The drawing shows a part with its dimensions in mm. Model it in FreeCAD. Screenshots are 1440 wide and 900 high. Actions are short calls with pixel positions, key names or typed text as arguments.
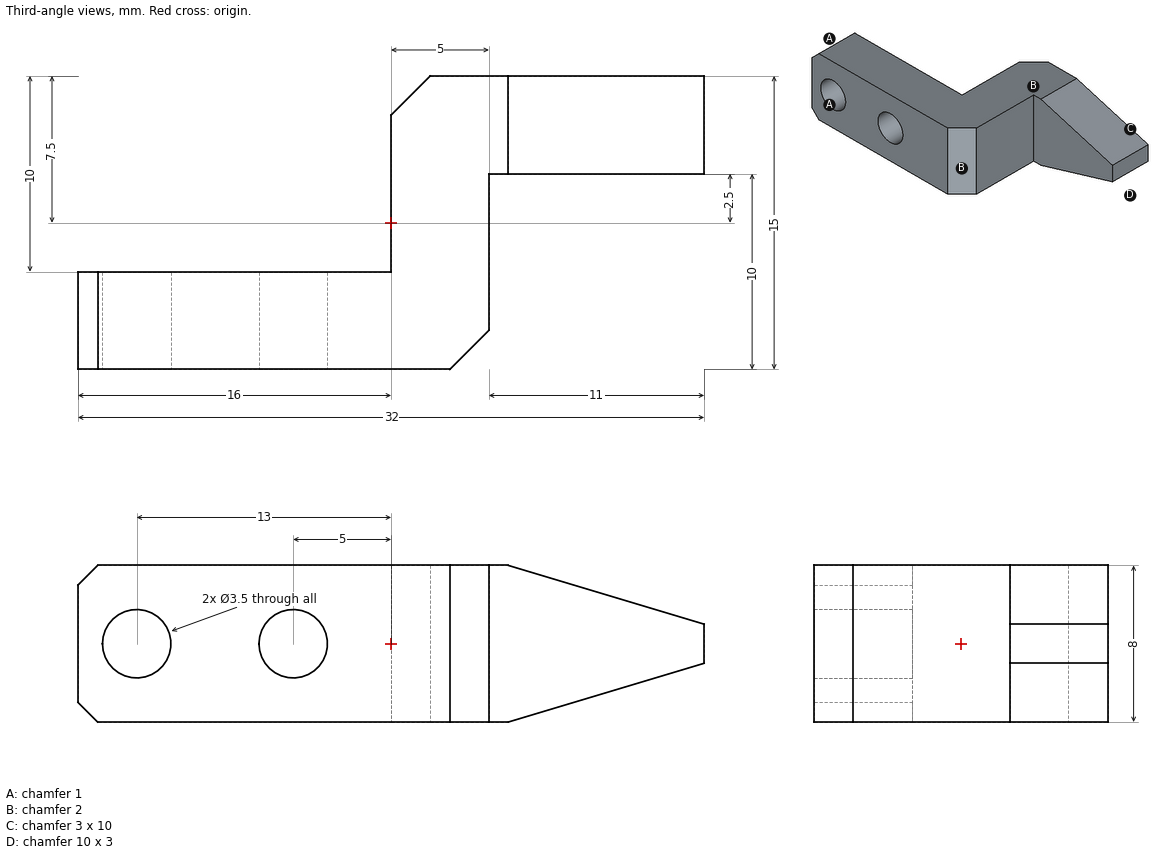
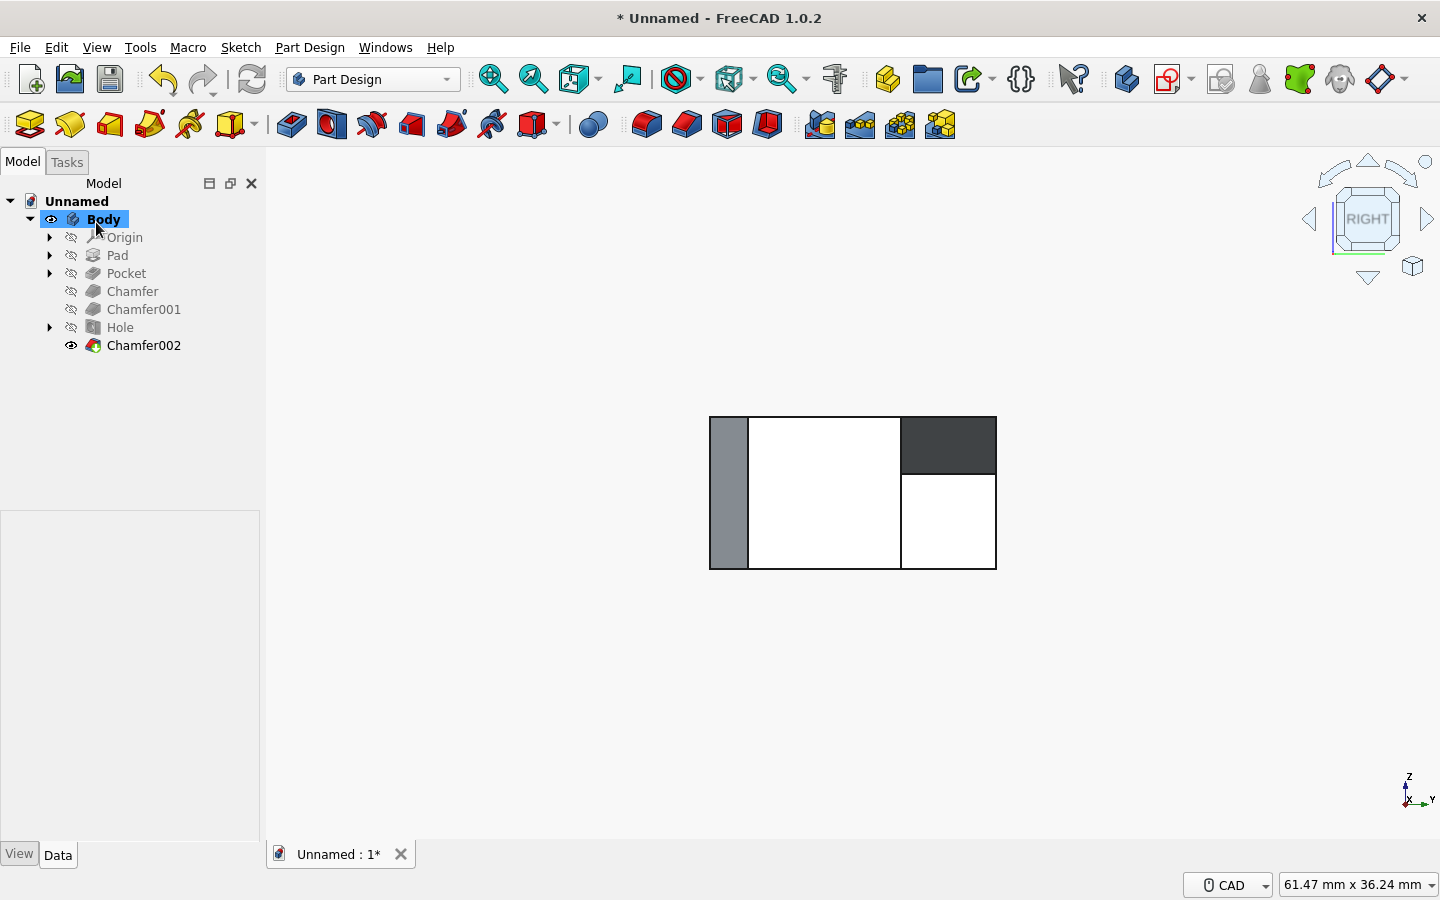
click(948, 568)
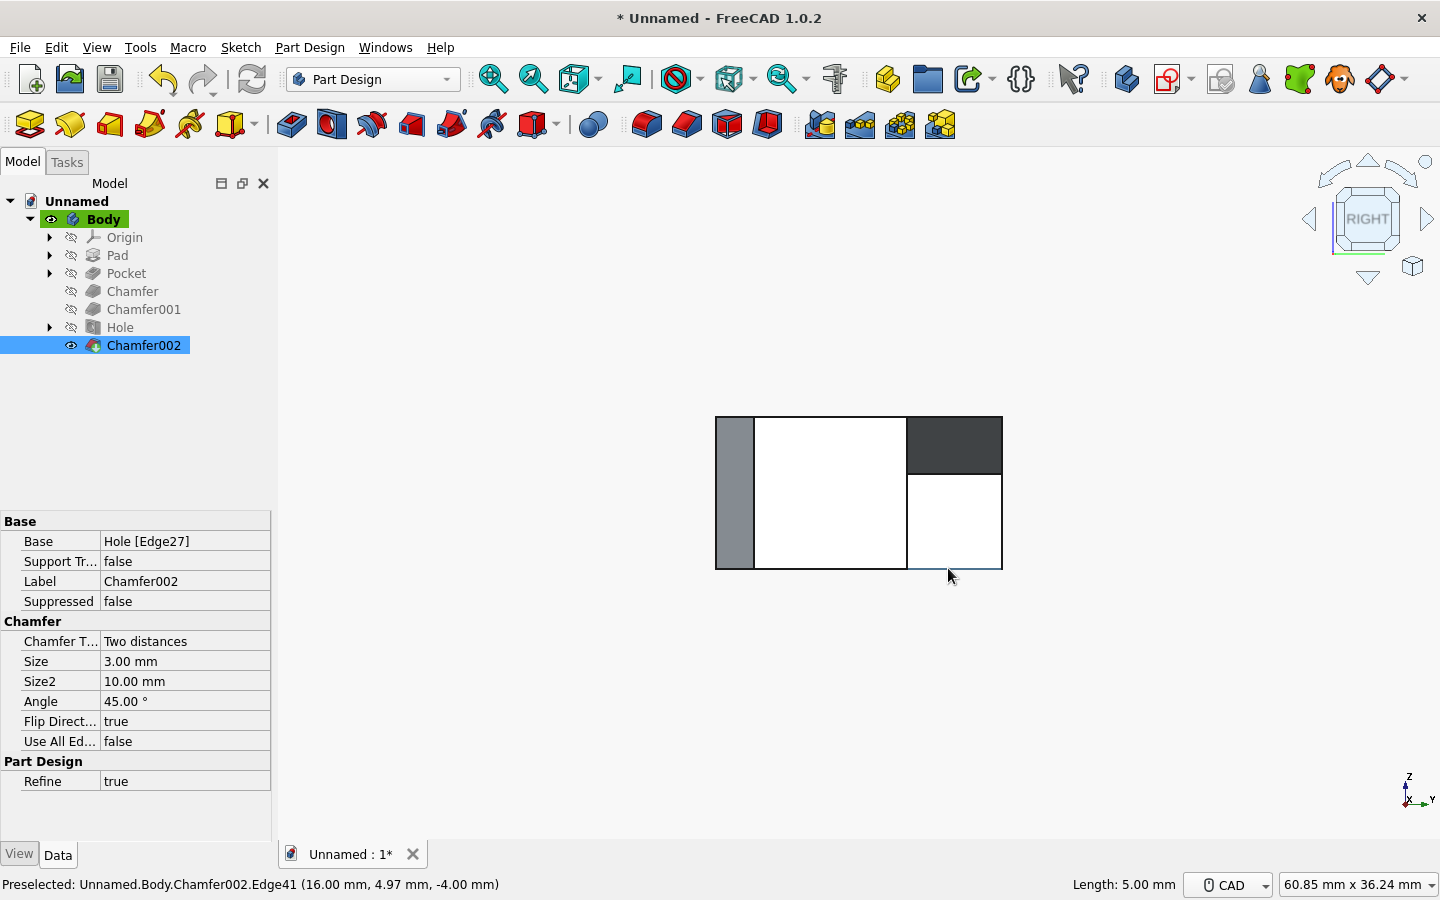
click(688, 124)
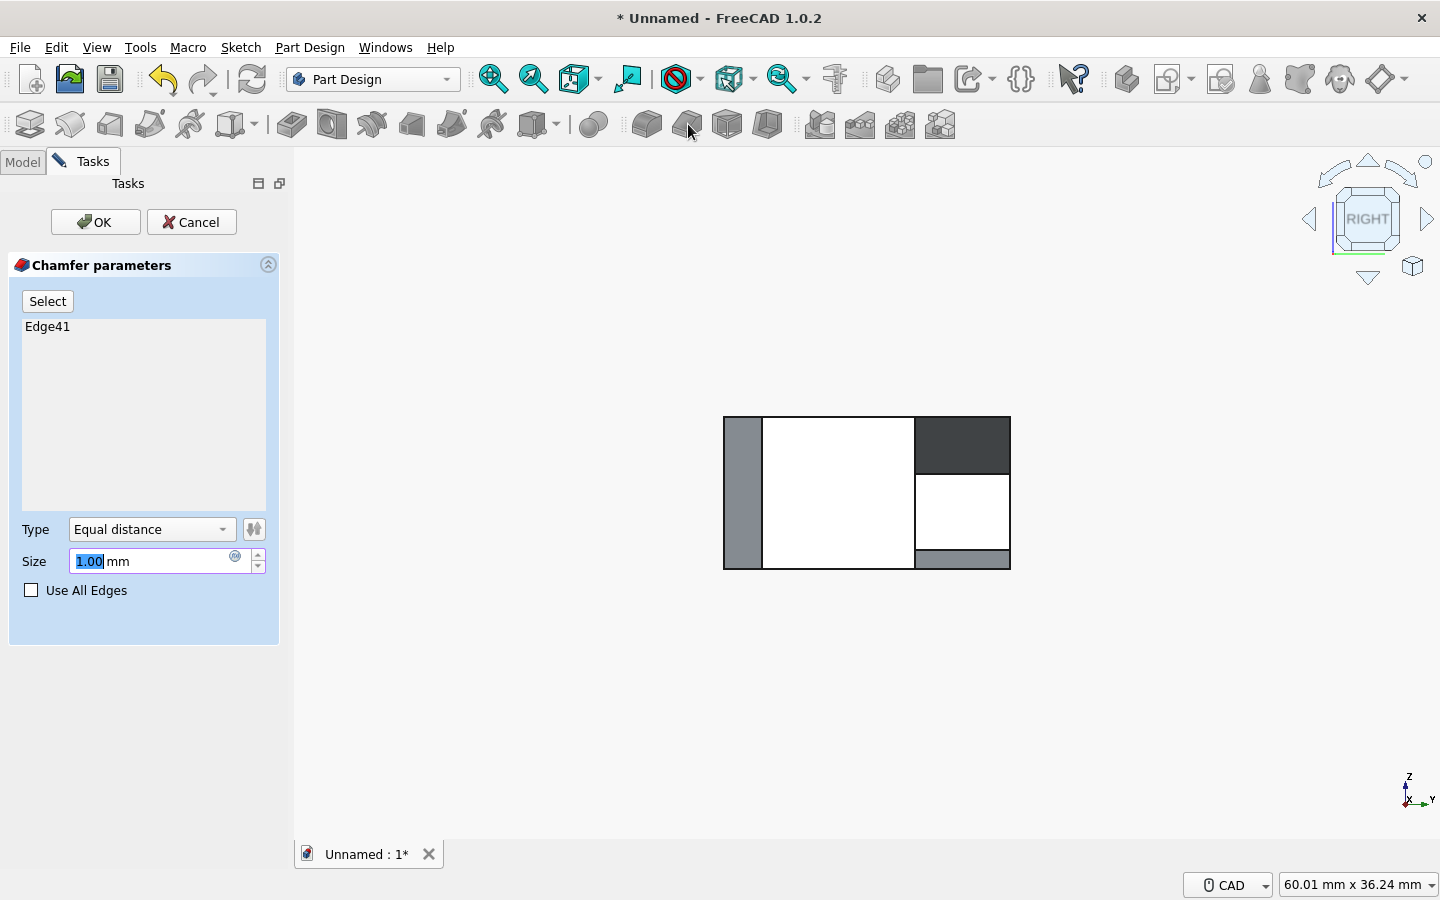
text(10)
key(Tab)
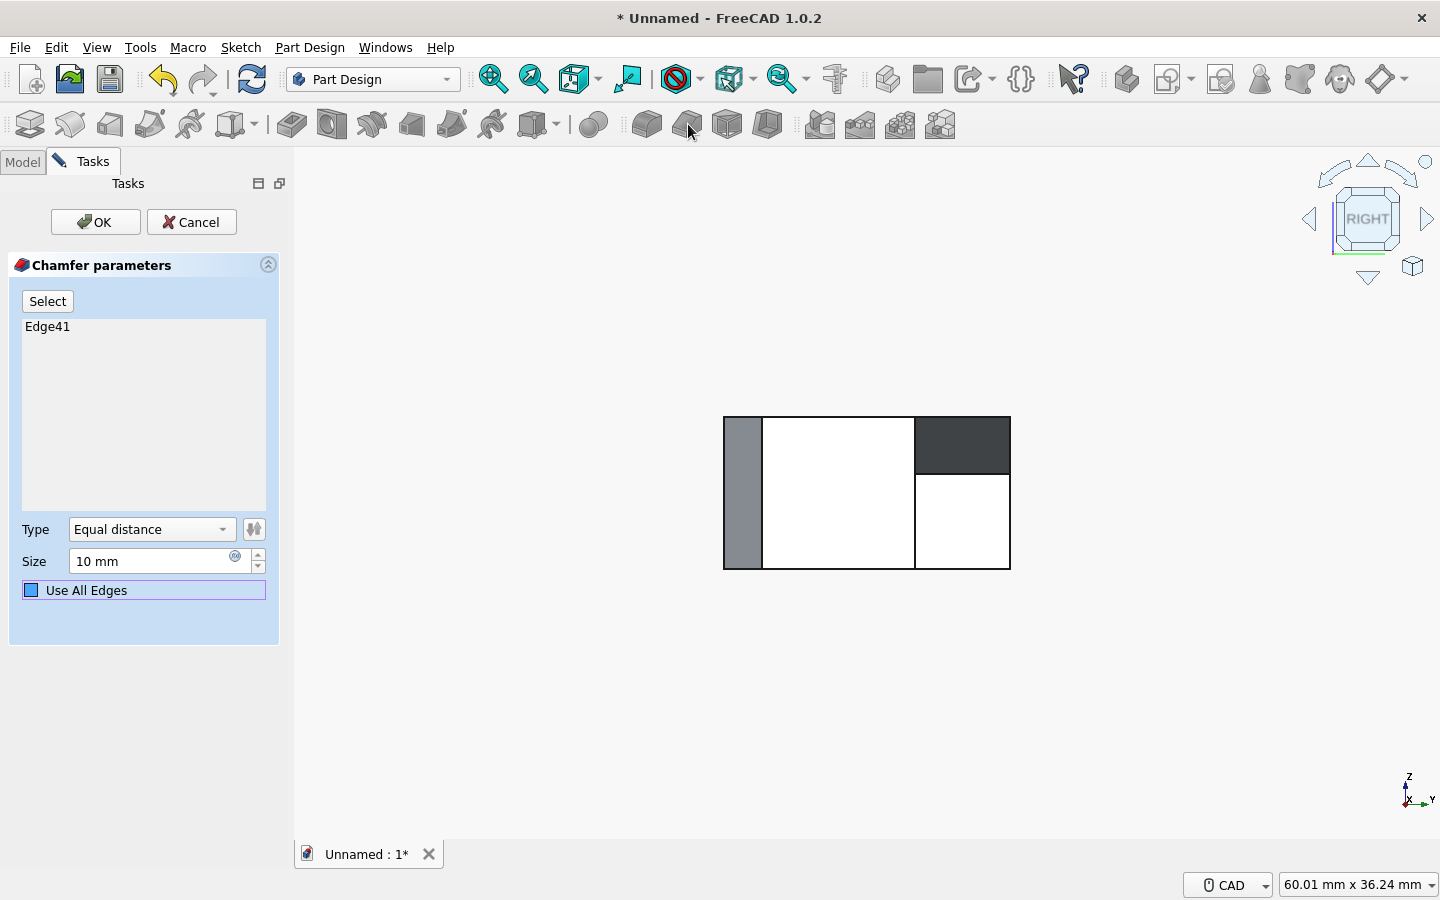
click(153, 530)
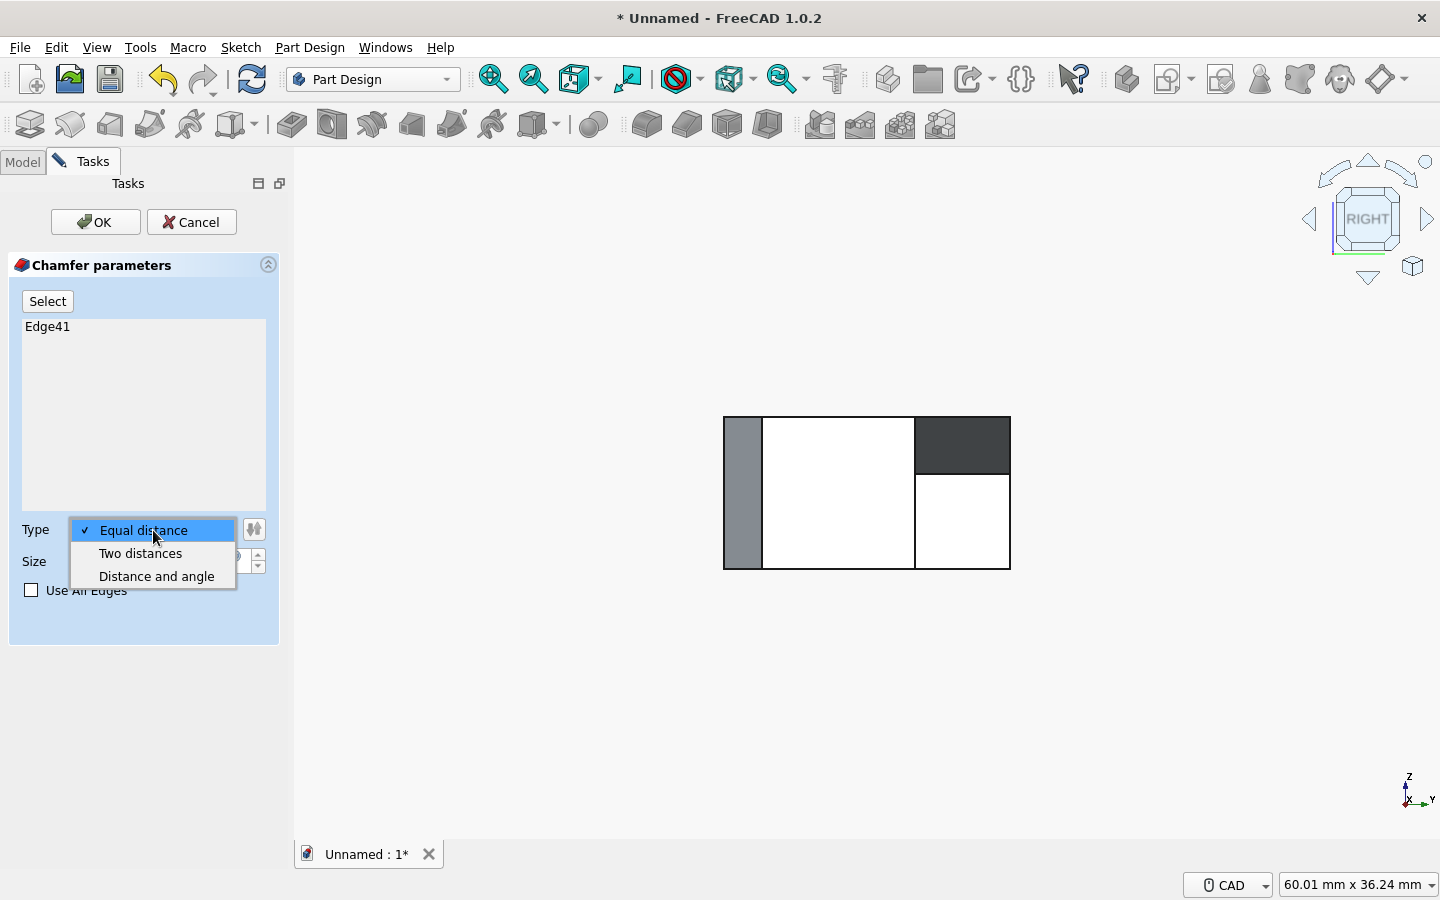
click(152, 554)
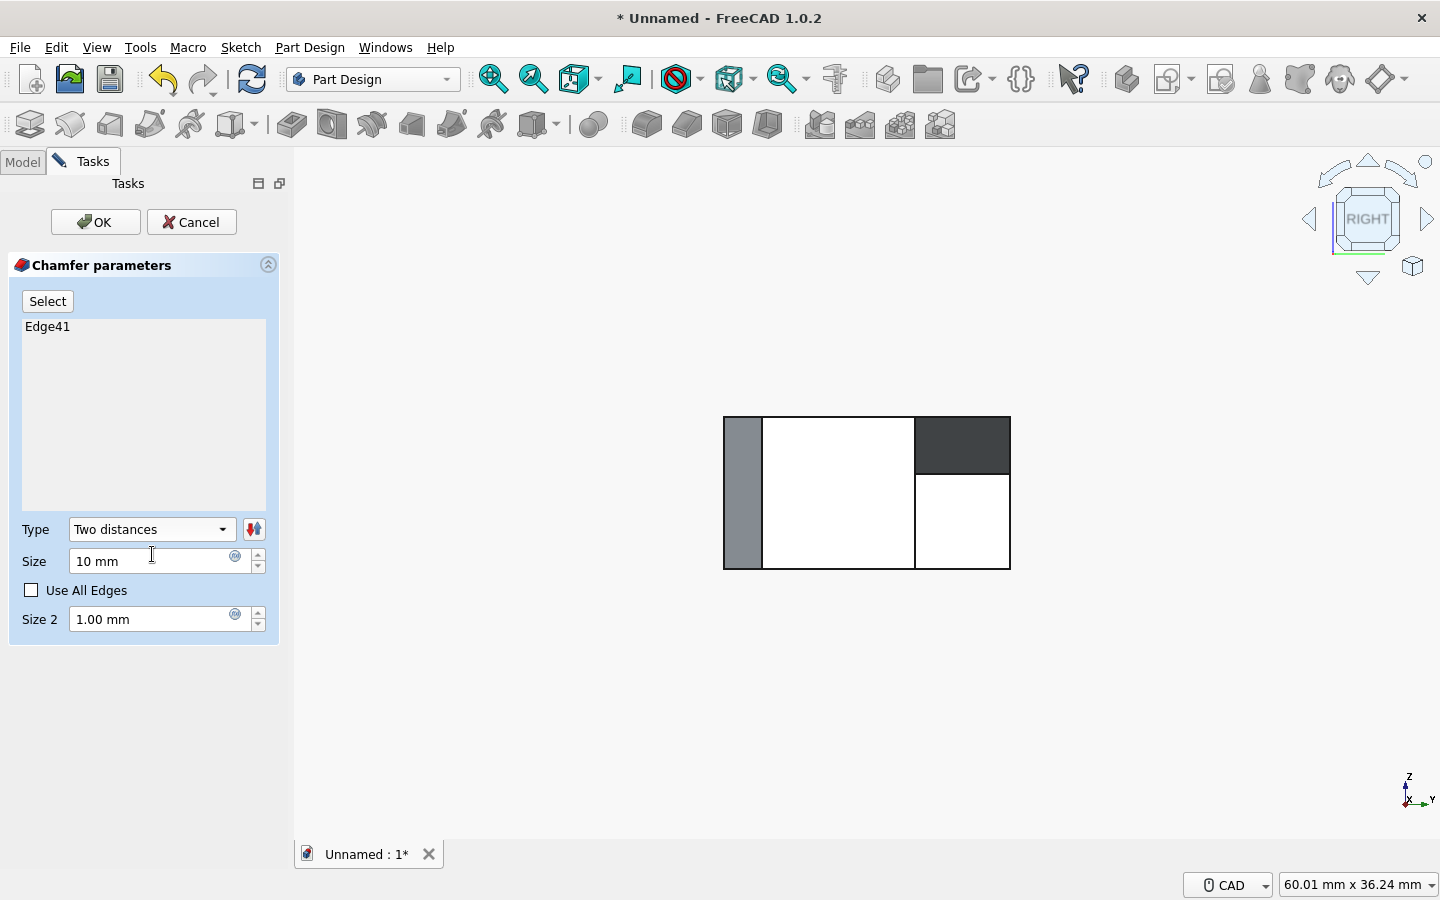
triple_click(160, 619)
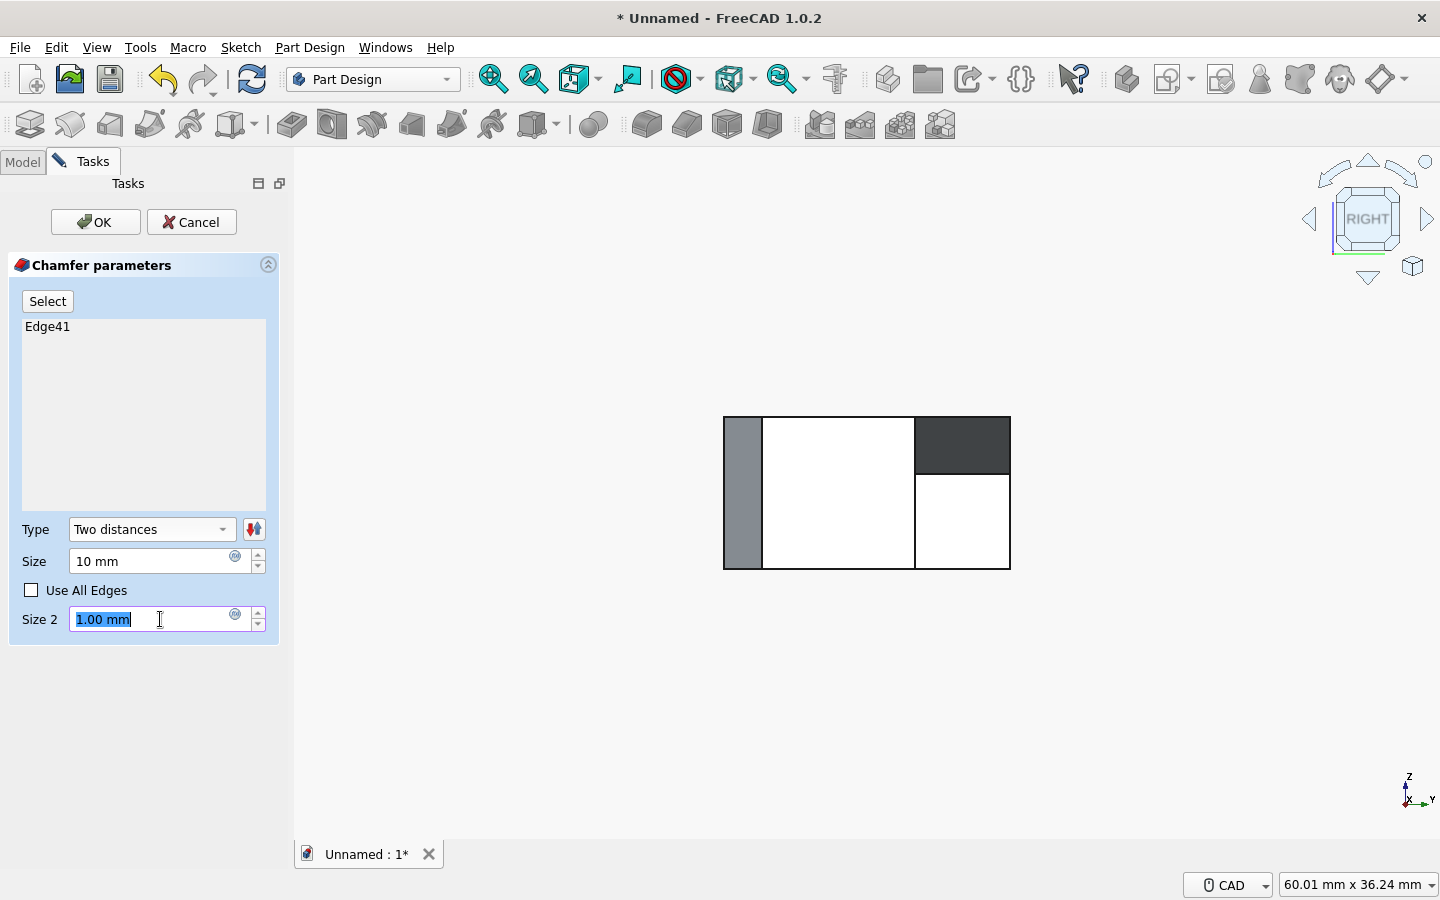
text(3)
key(Tab)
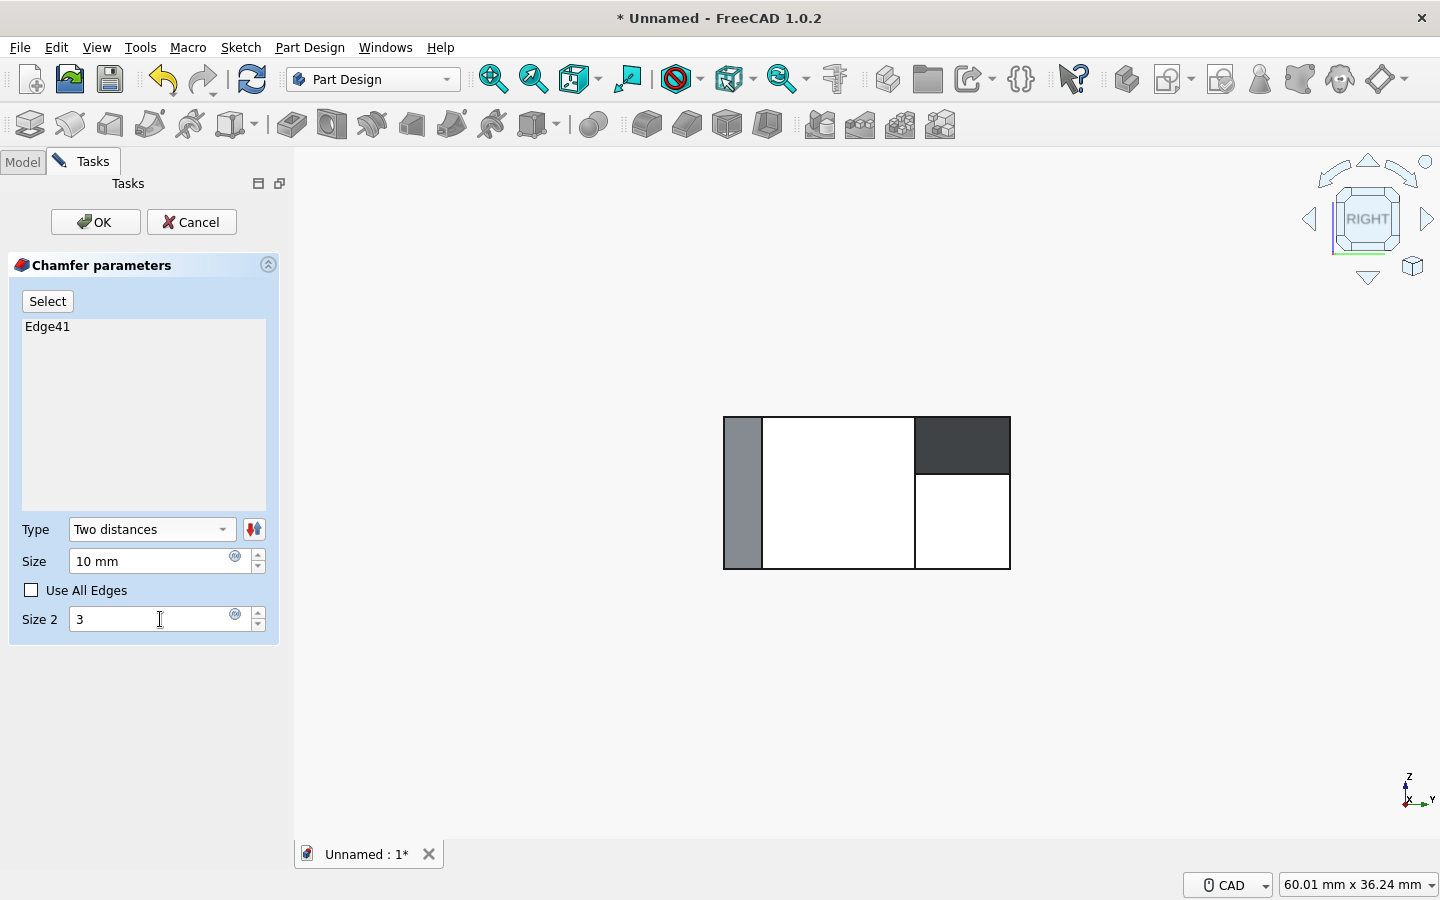
click(254, 530)